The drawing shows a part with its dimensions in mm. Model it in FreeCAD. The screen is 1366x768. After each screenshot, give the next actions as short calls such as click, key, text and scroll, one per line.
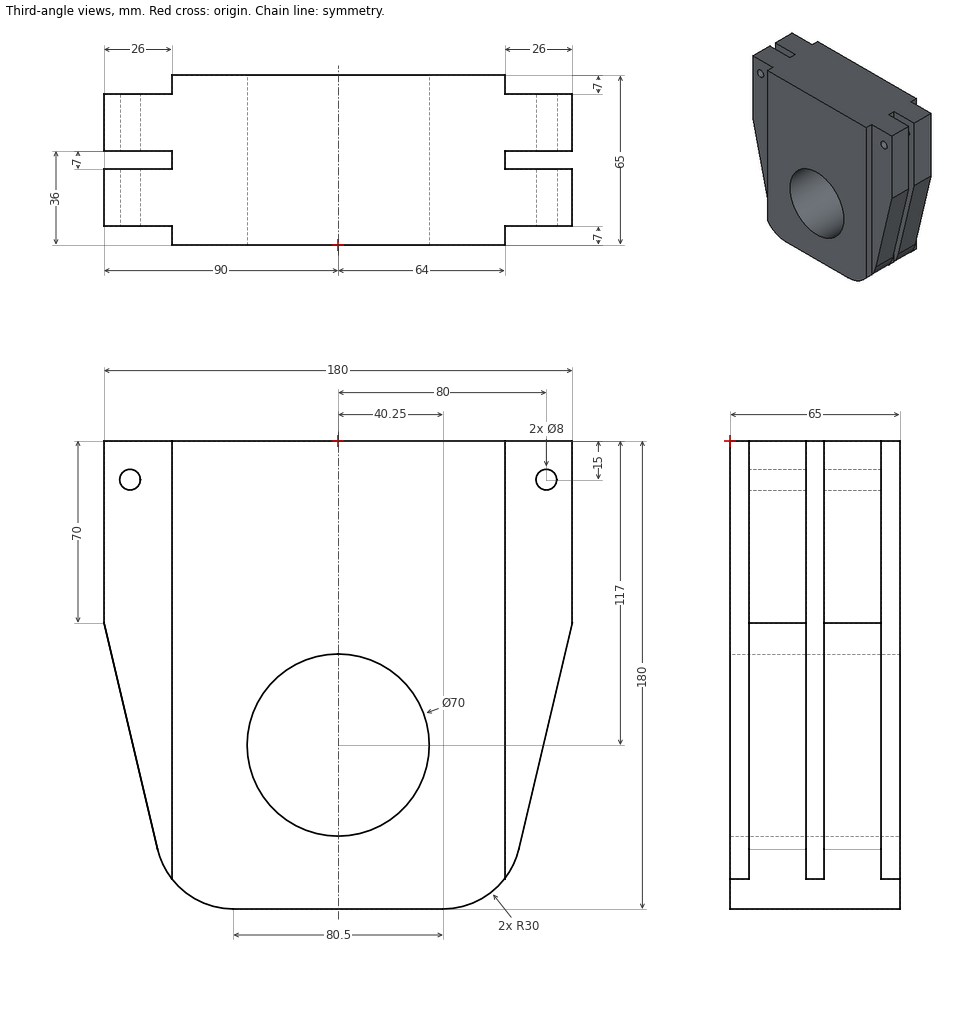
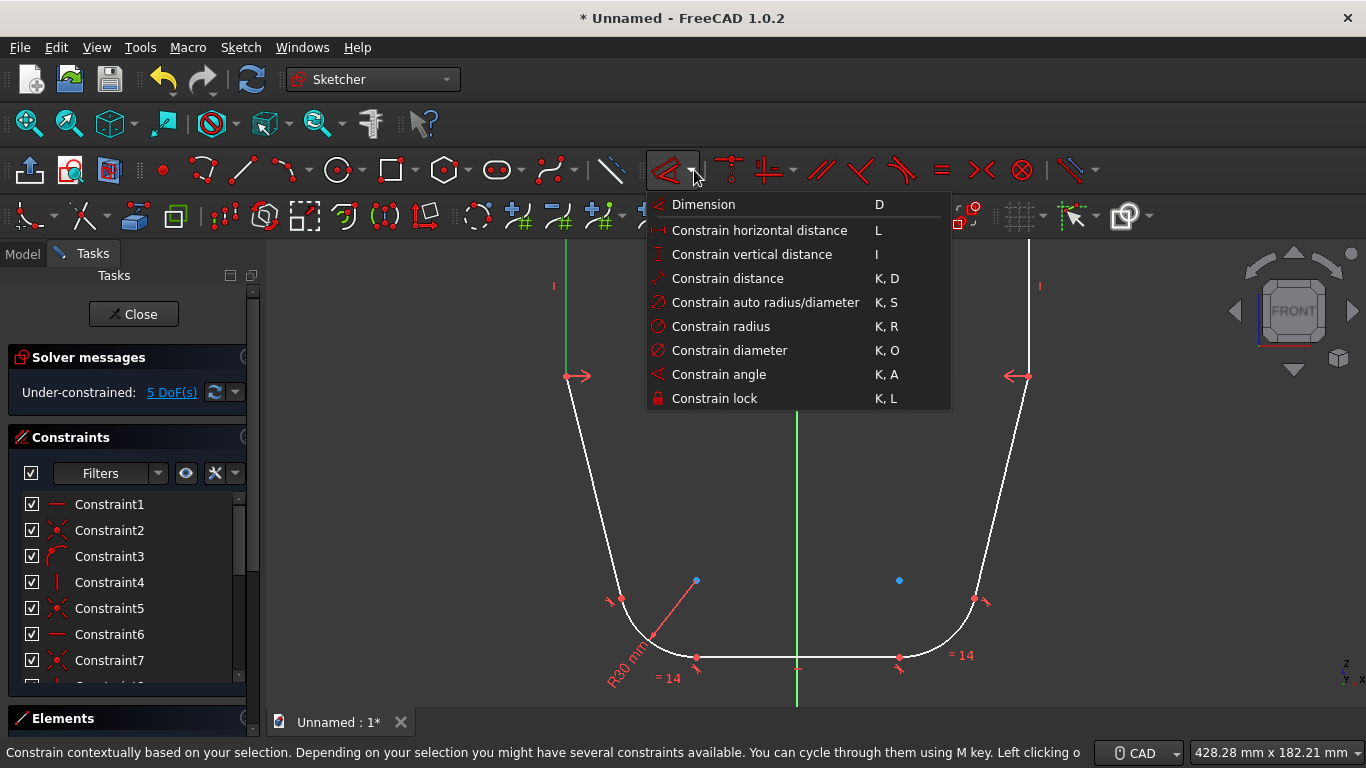
click(799, 254)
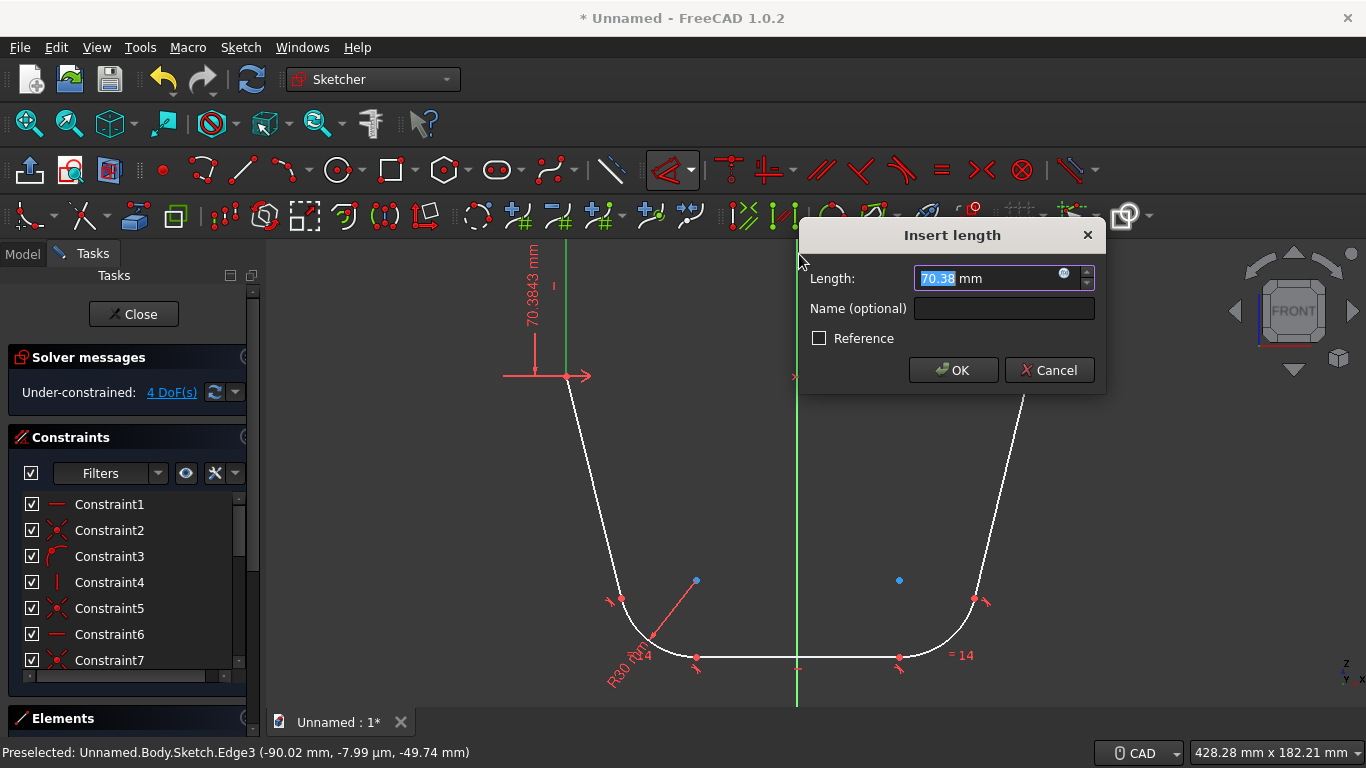
text(70)
key(Return)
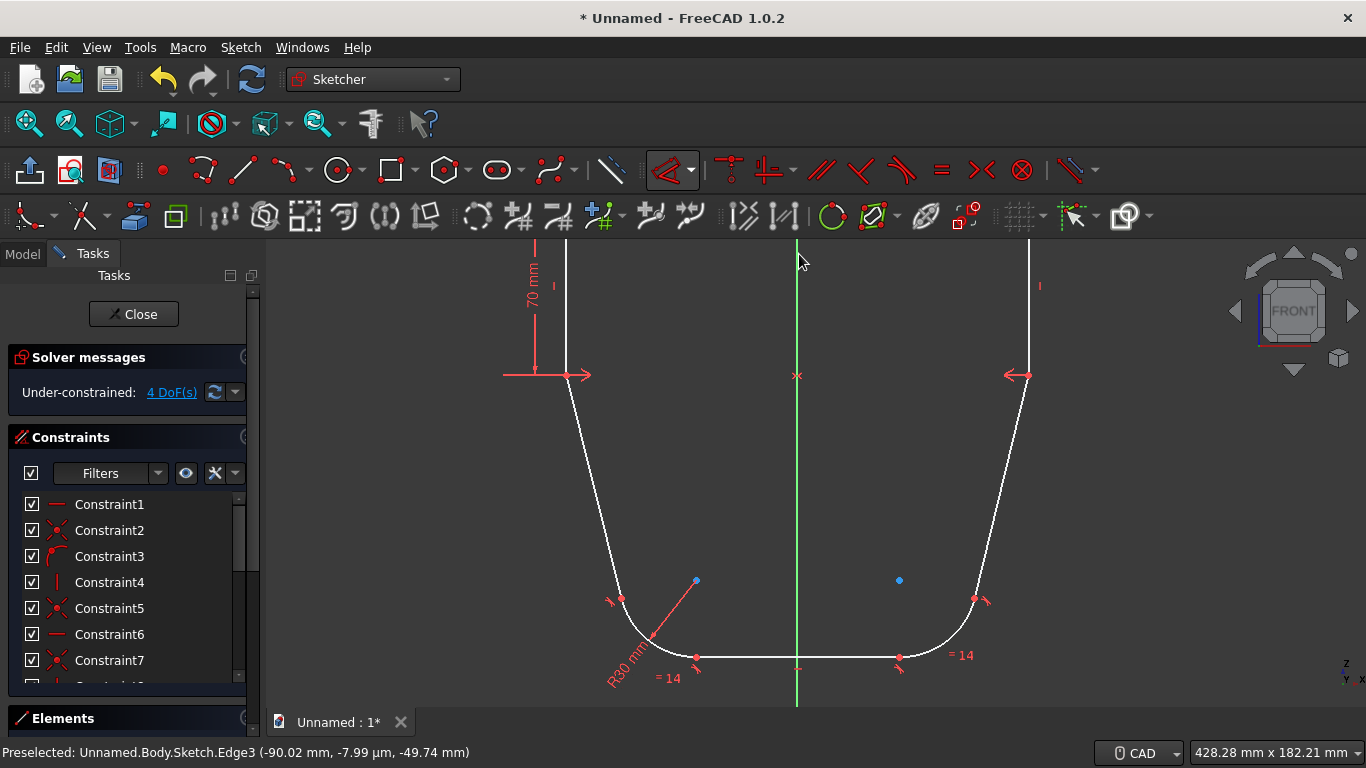
scroll(646, 568, down, 2)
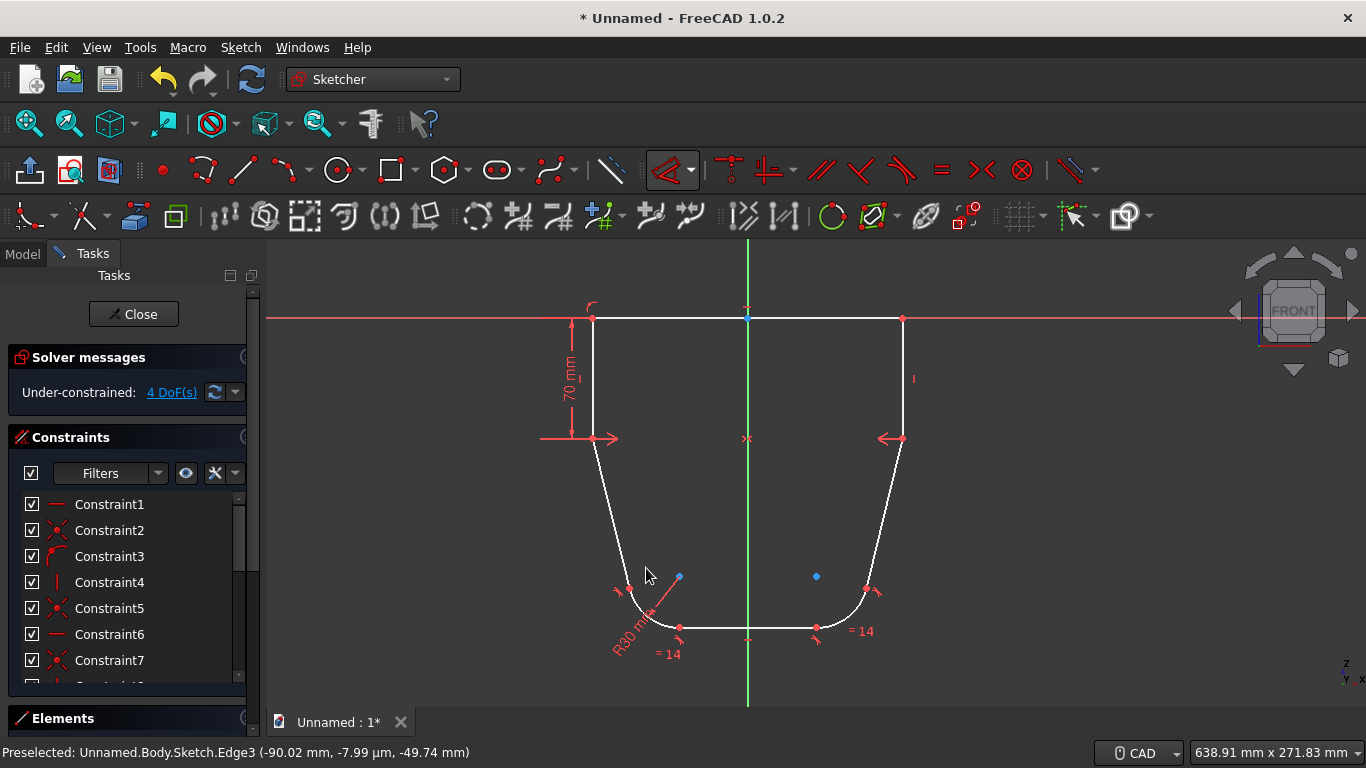
click(686, 318)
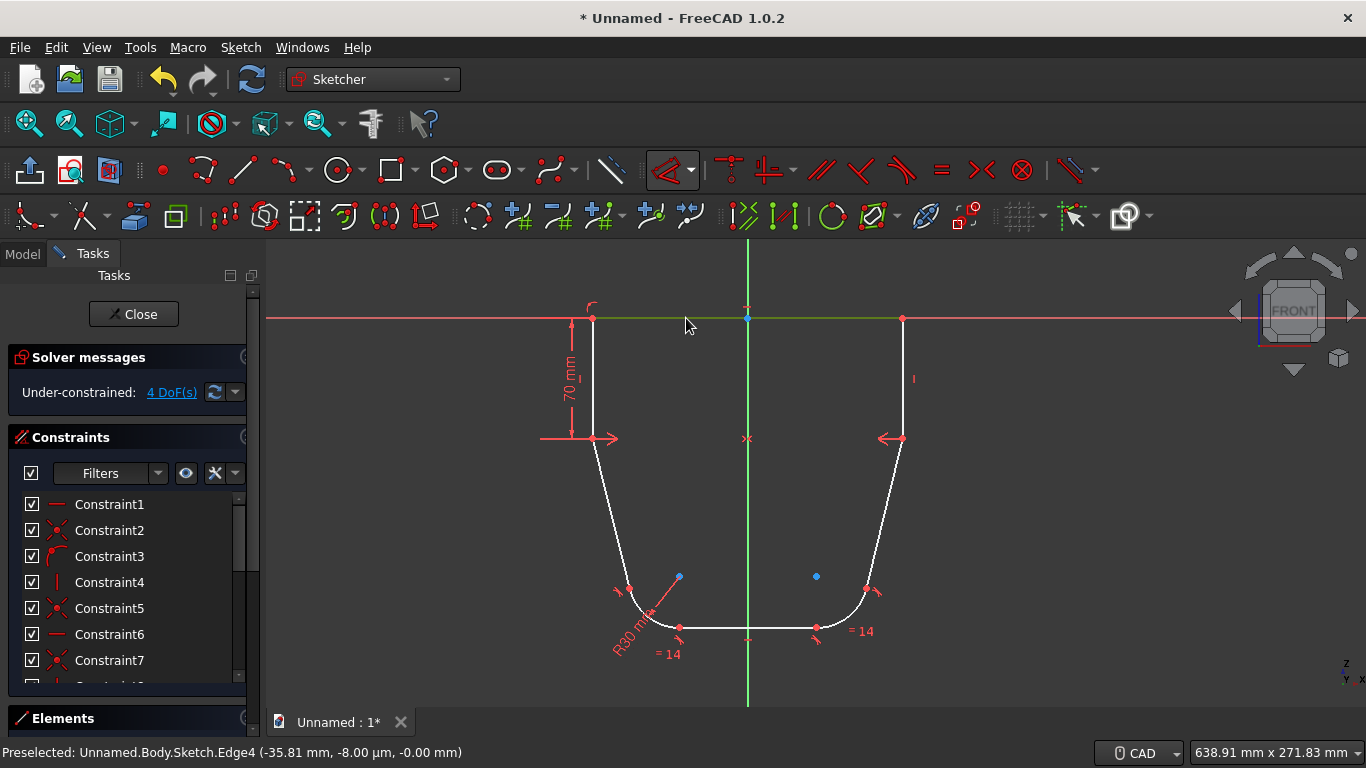
click(694, 170)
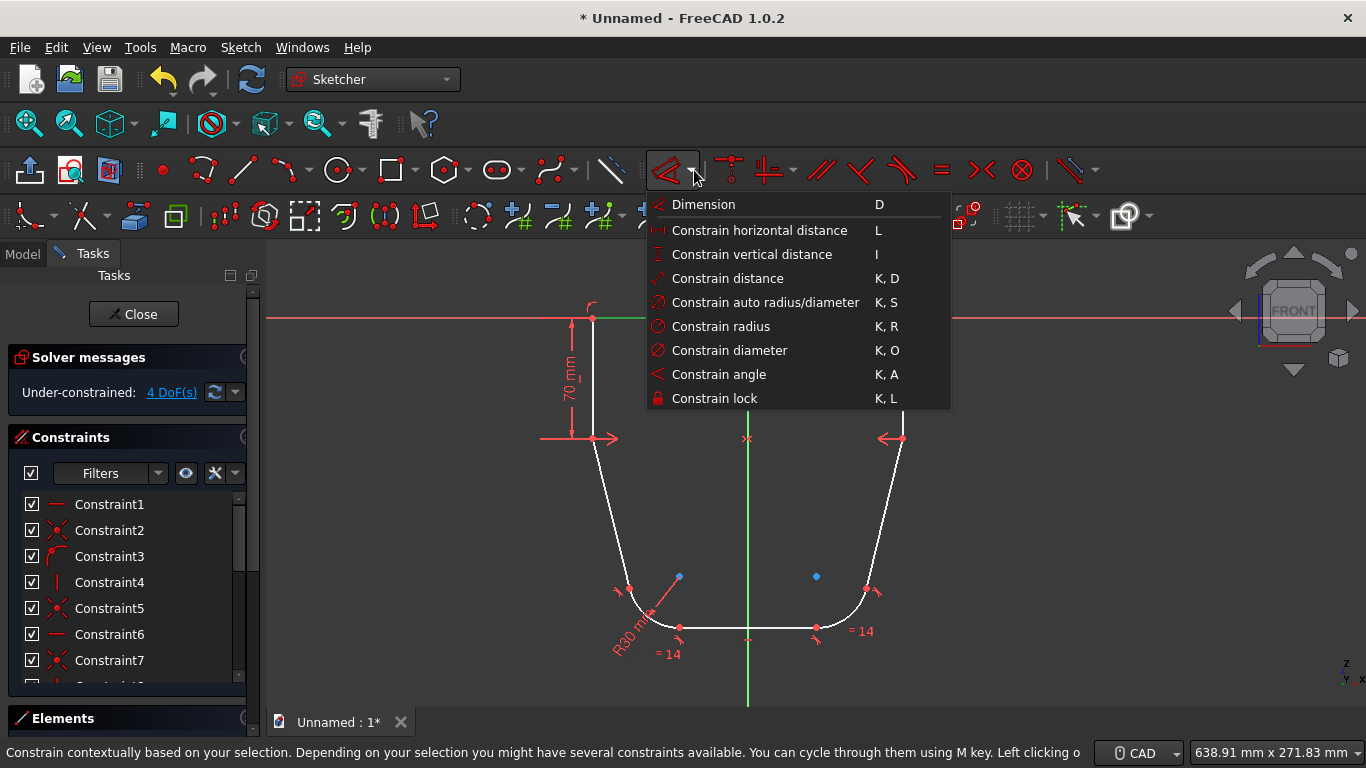
click(799, 230)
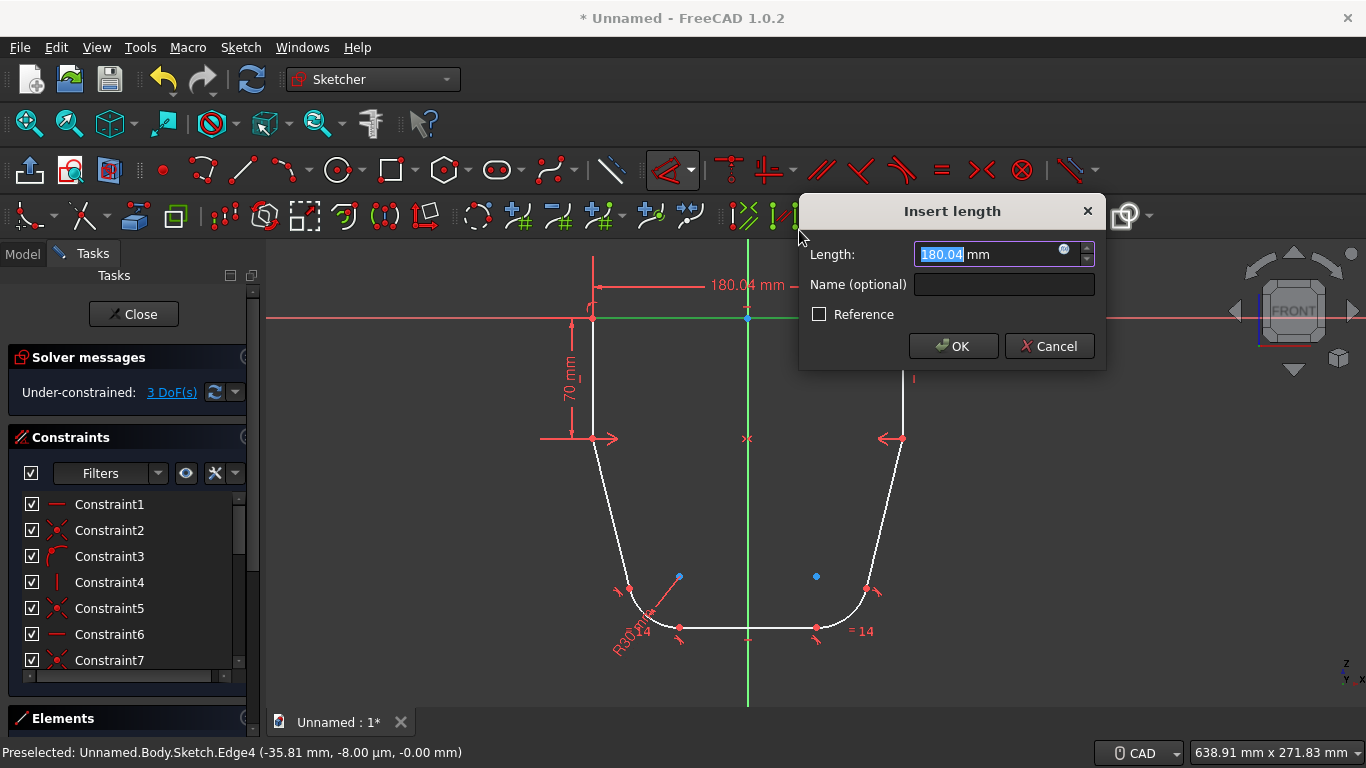
text(180)
key(Return)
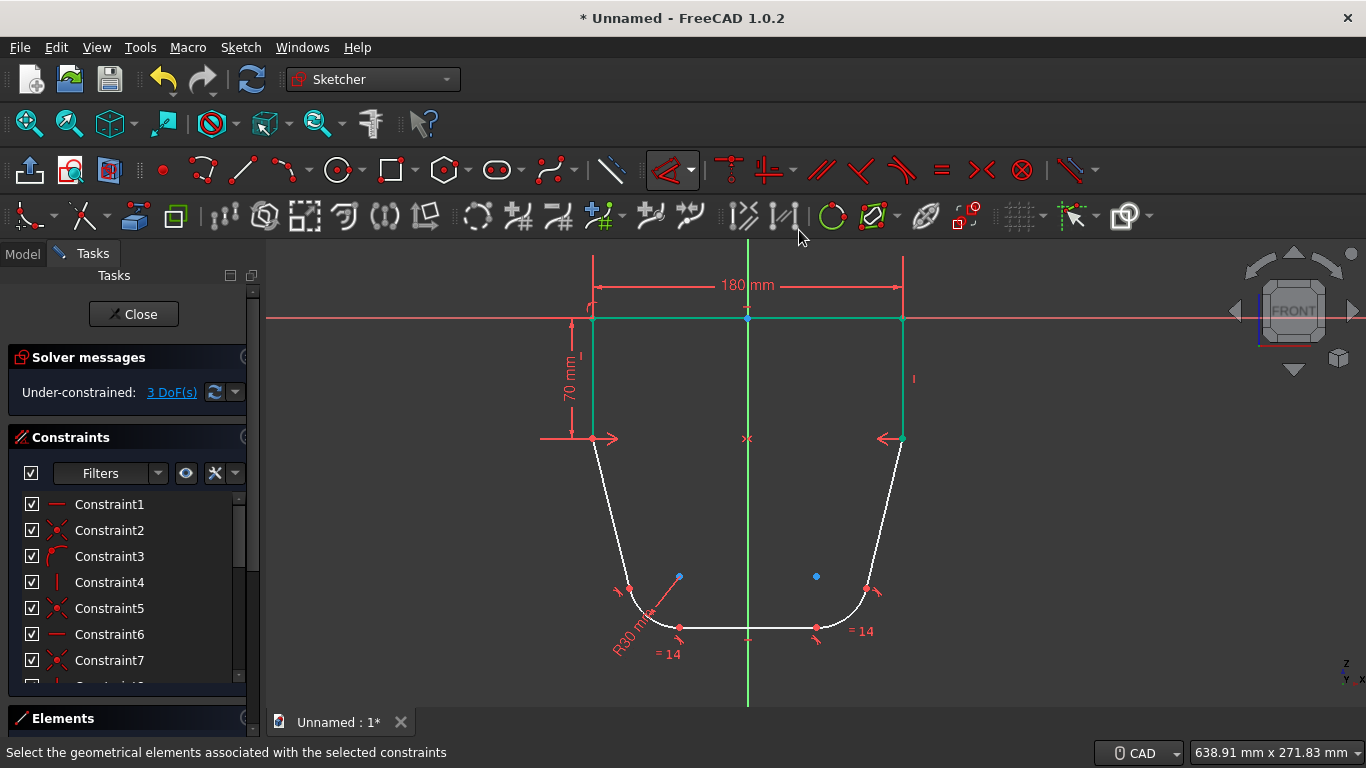
click(775, 628)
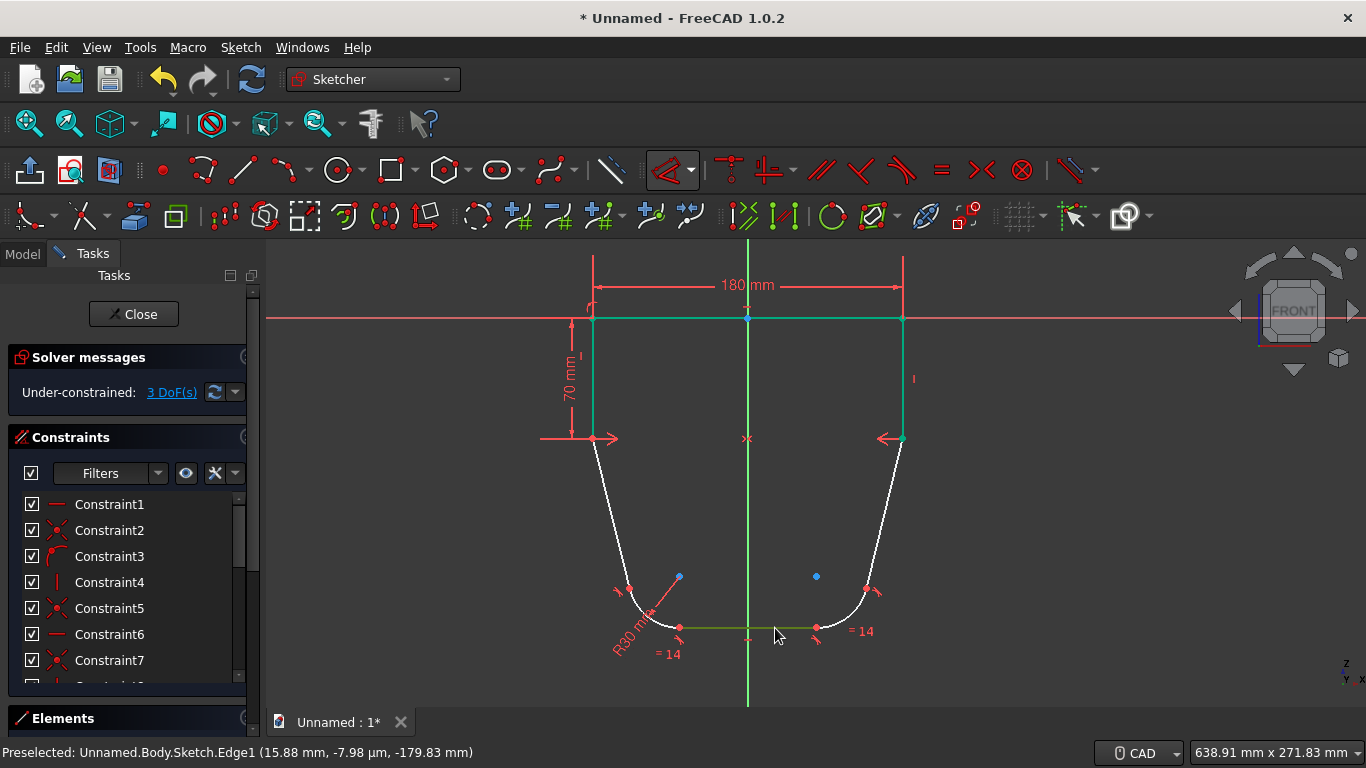
key(l)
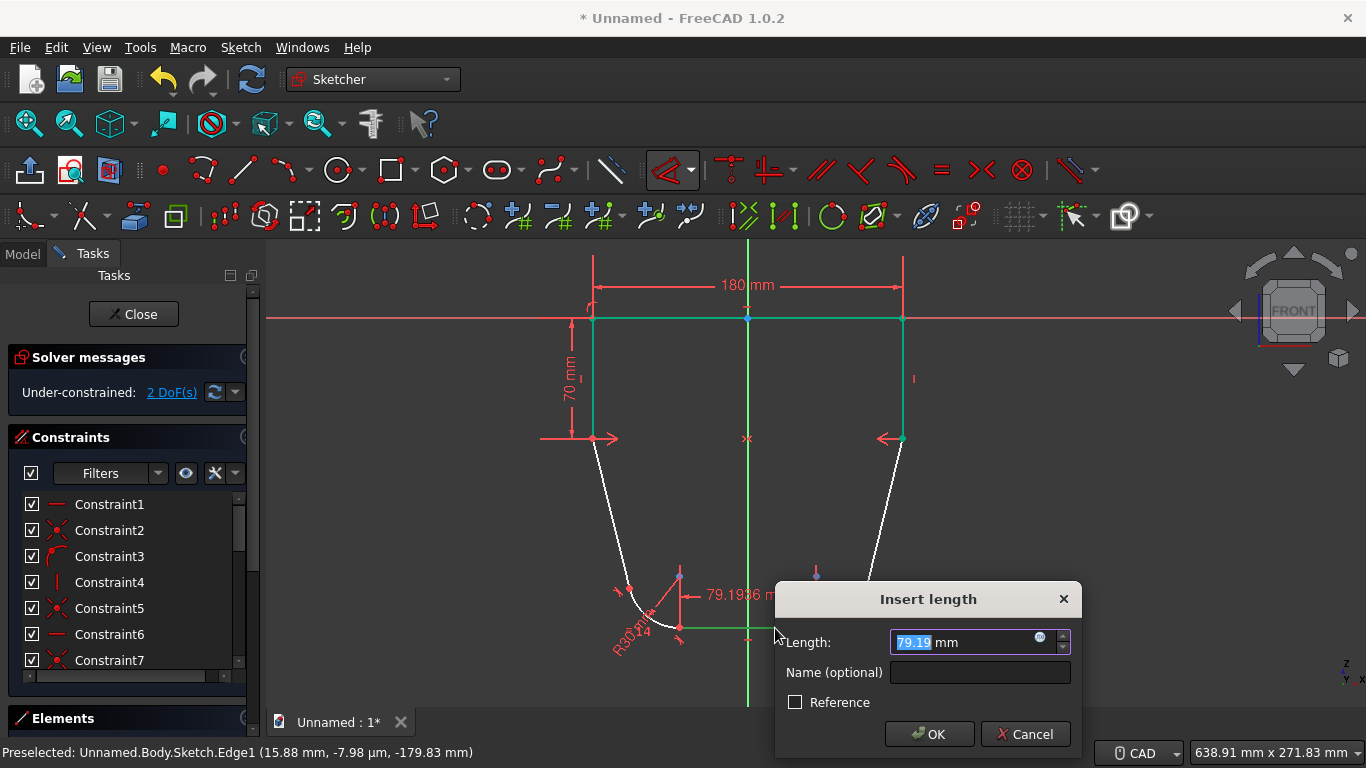
text(80.5)
key(Return)